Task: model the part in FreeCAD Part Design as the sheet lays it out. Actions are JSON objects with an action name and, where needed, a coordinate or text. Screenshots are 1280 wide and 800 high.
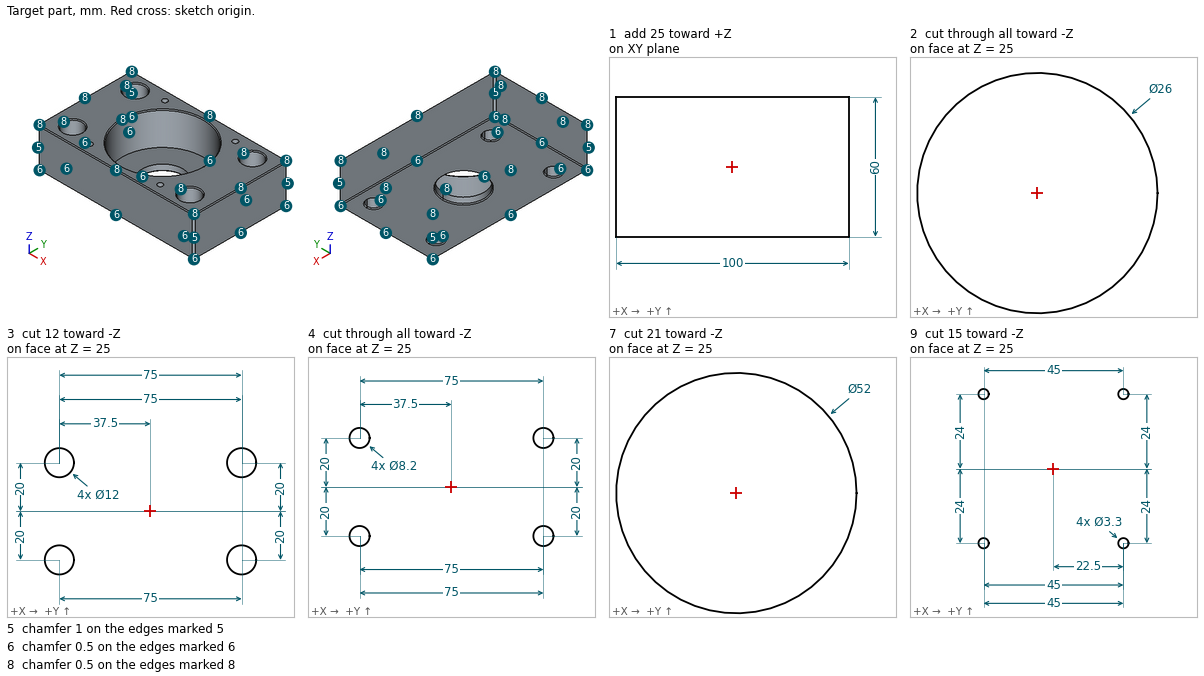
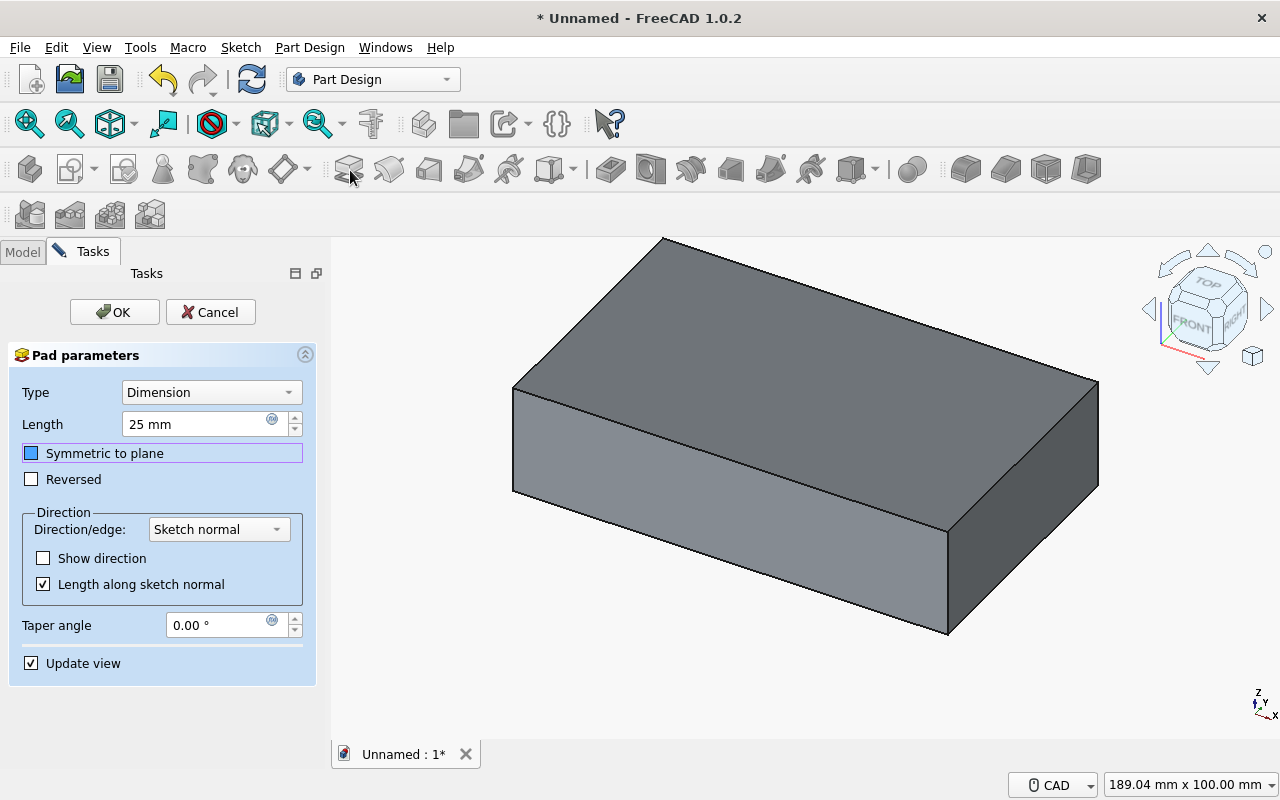
{"action": "left_click", "coordinate": [115, 312]}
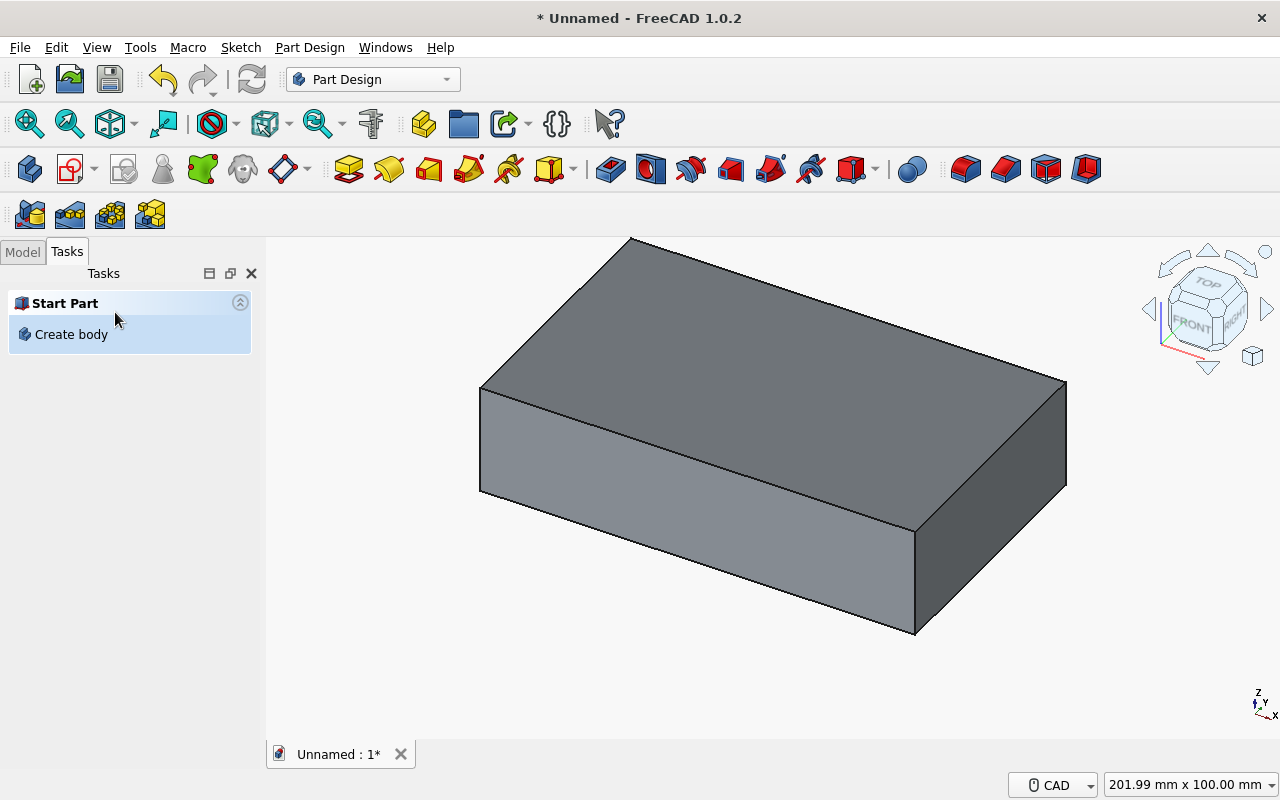
{"action": "left_click", "coordinate": [835, 405]}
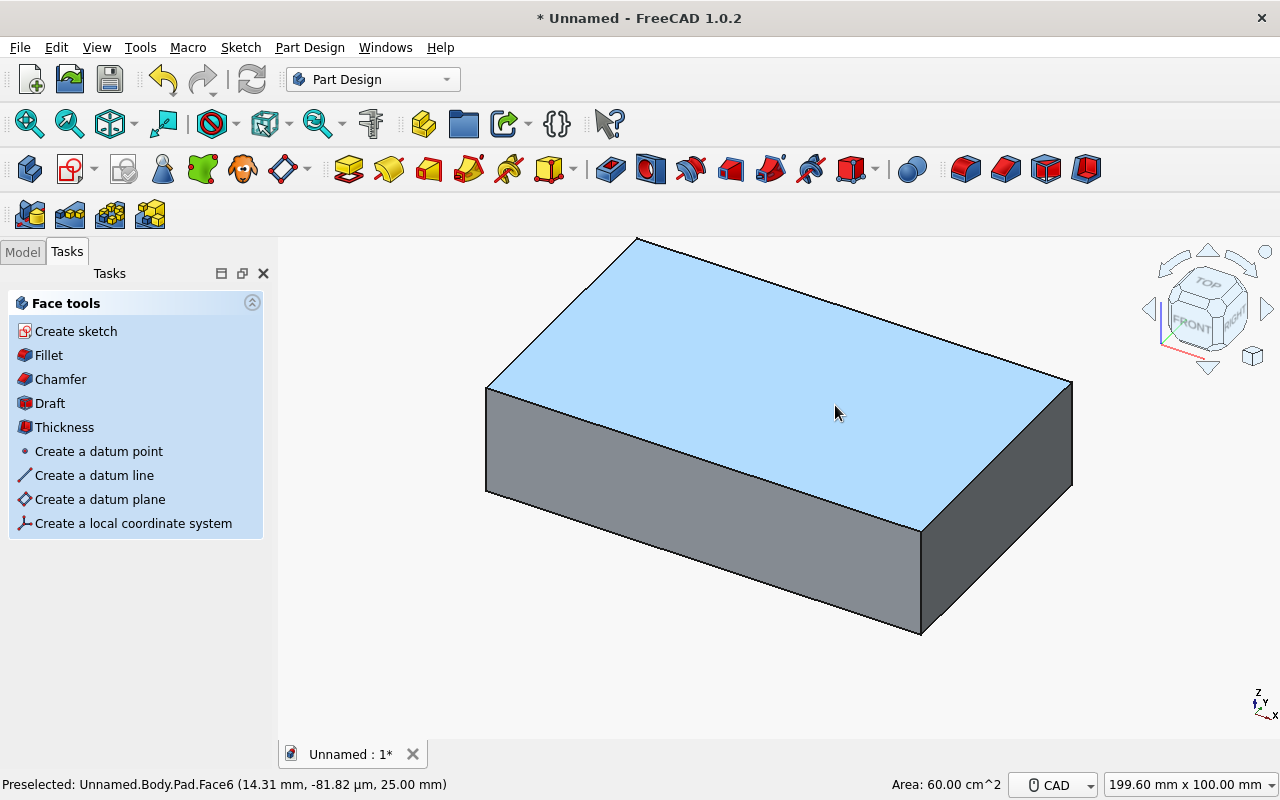
{"action": "left_click", "coordinate": [70, 170]}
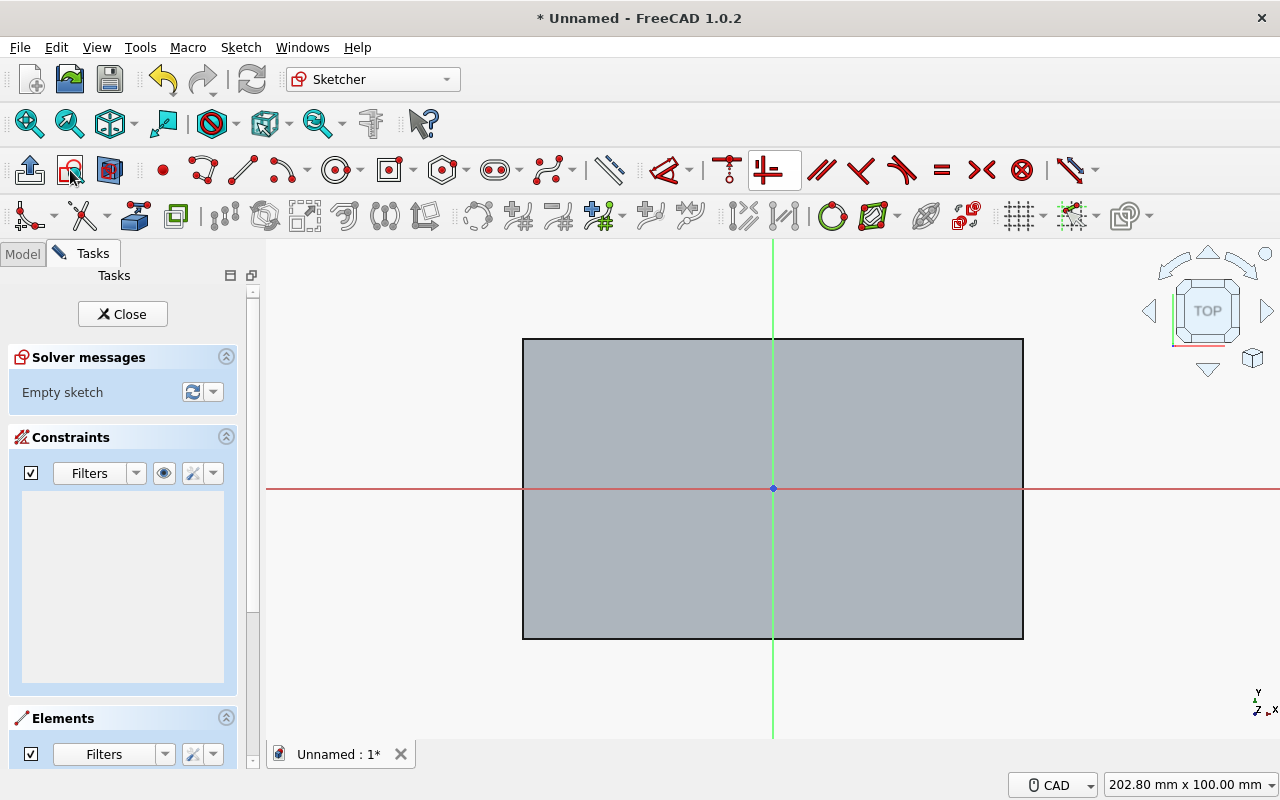
{"action": "scroll", "coordinate": [829, 489], "scroll_direction": "up", "scroll_amount": 4}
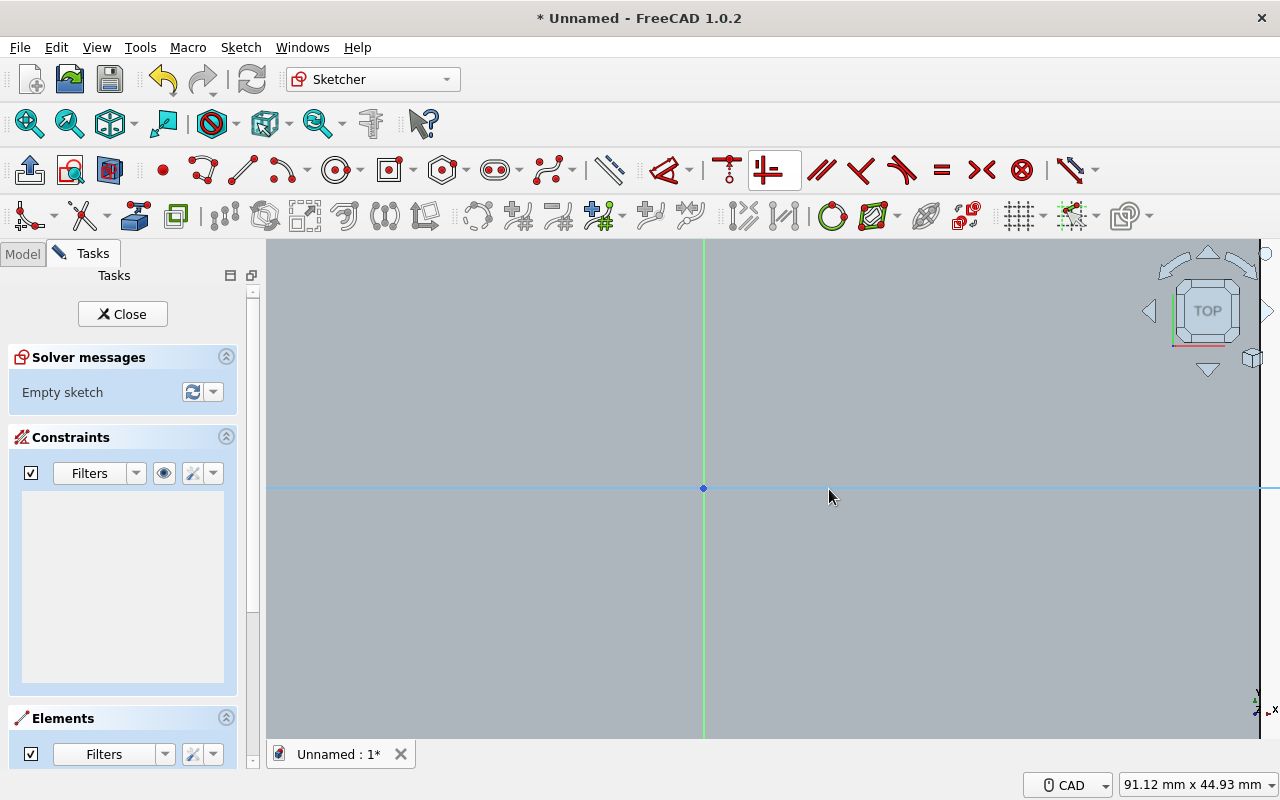
{"action": "left_click", "coordinate": [336, 170]}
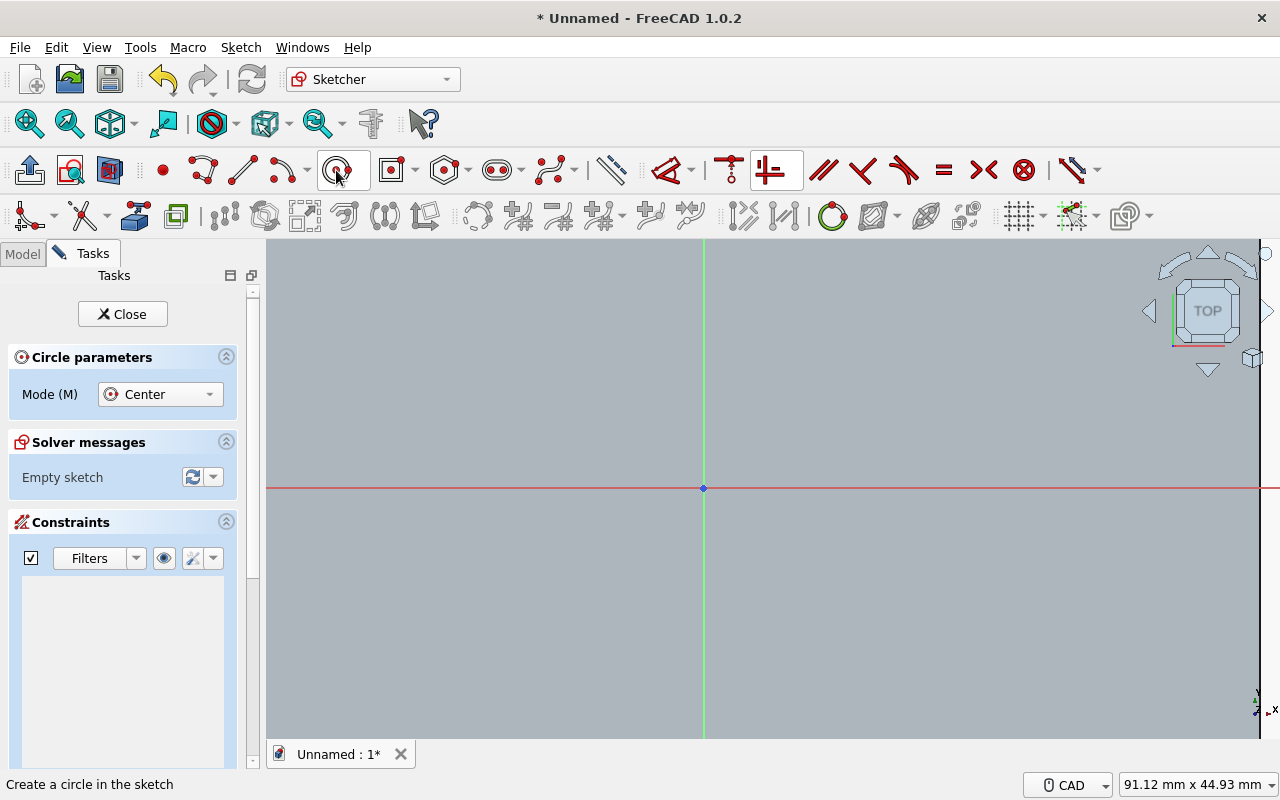
{"action": "left_click", "coordinate": [704, 488]}
{"action": "mouse_move", "coordinate": [806, 386]}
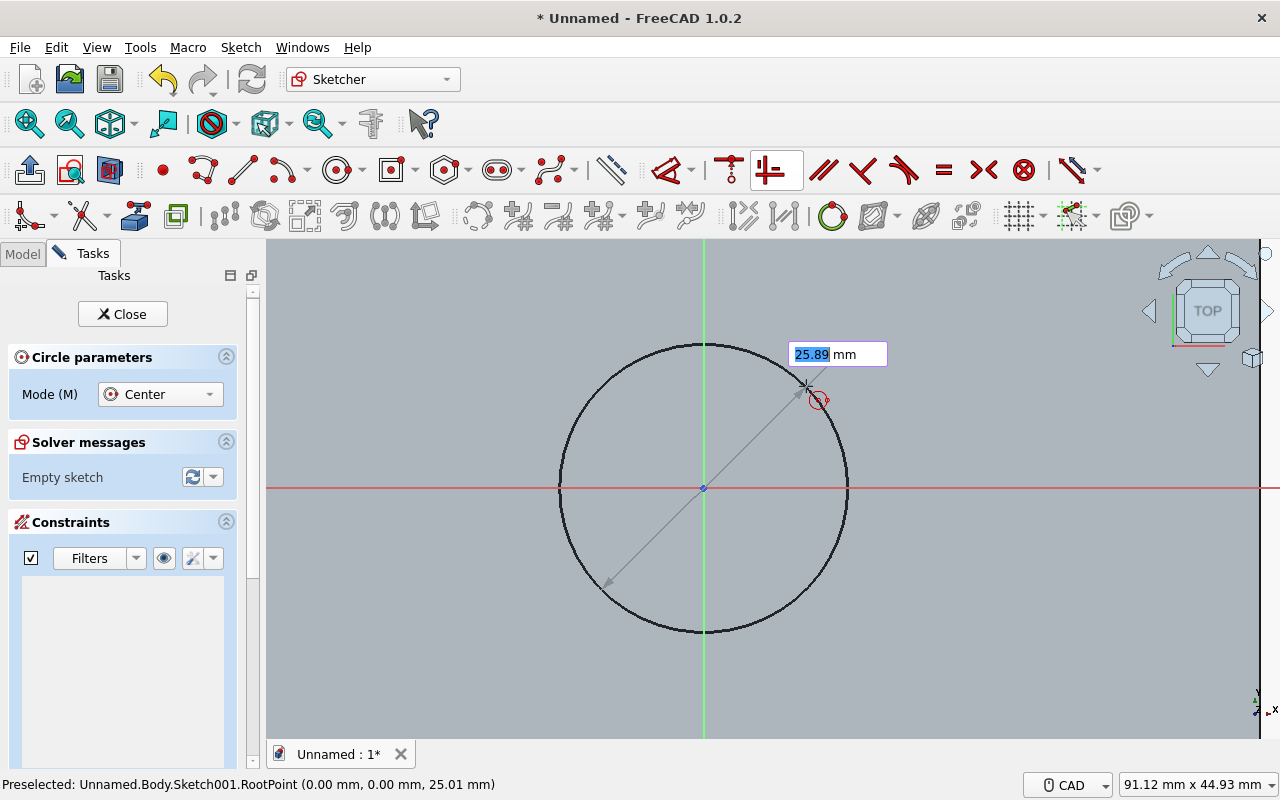
{"action": "type", "text": "26"}
{"action": "key", "text": "Return"}
{"action": "key", "text": "Escape"}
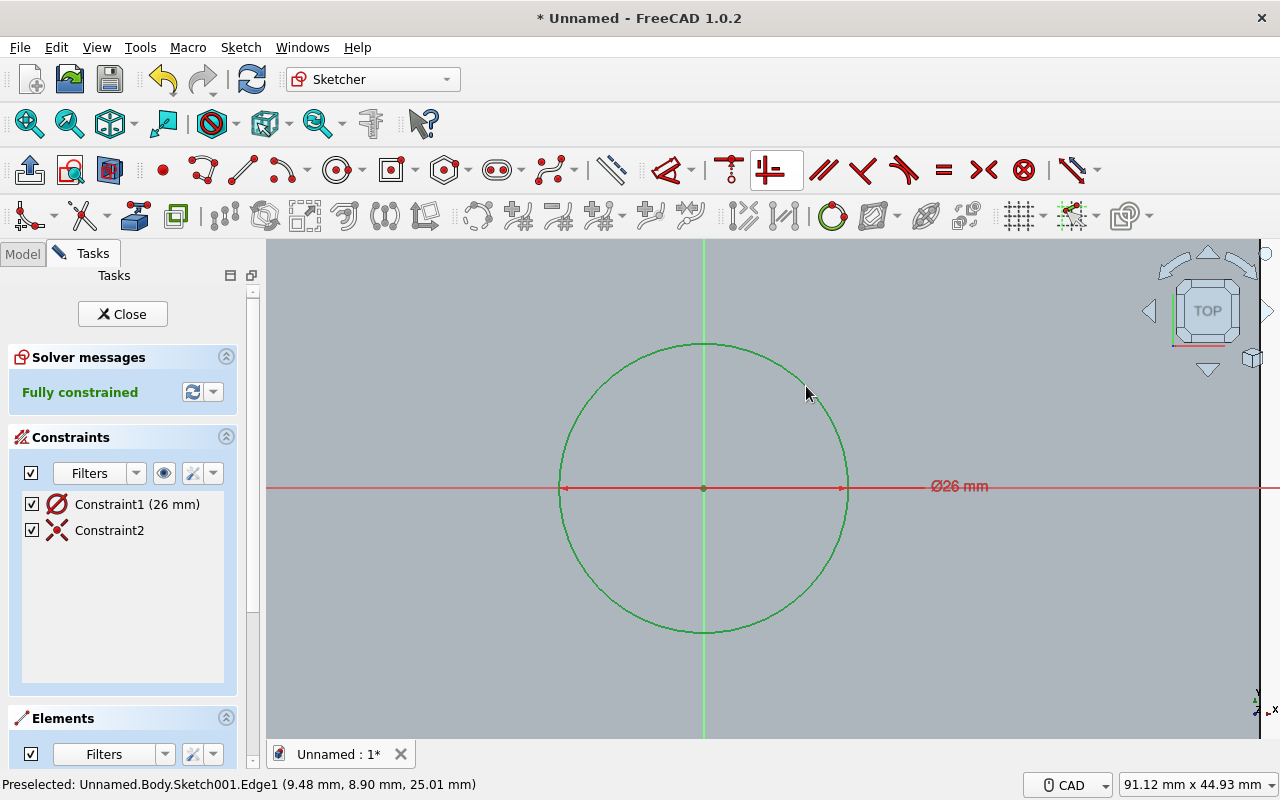
{"action": "left_click", "coordinate": [123, 314]}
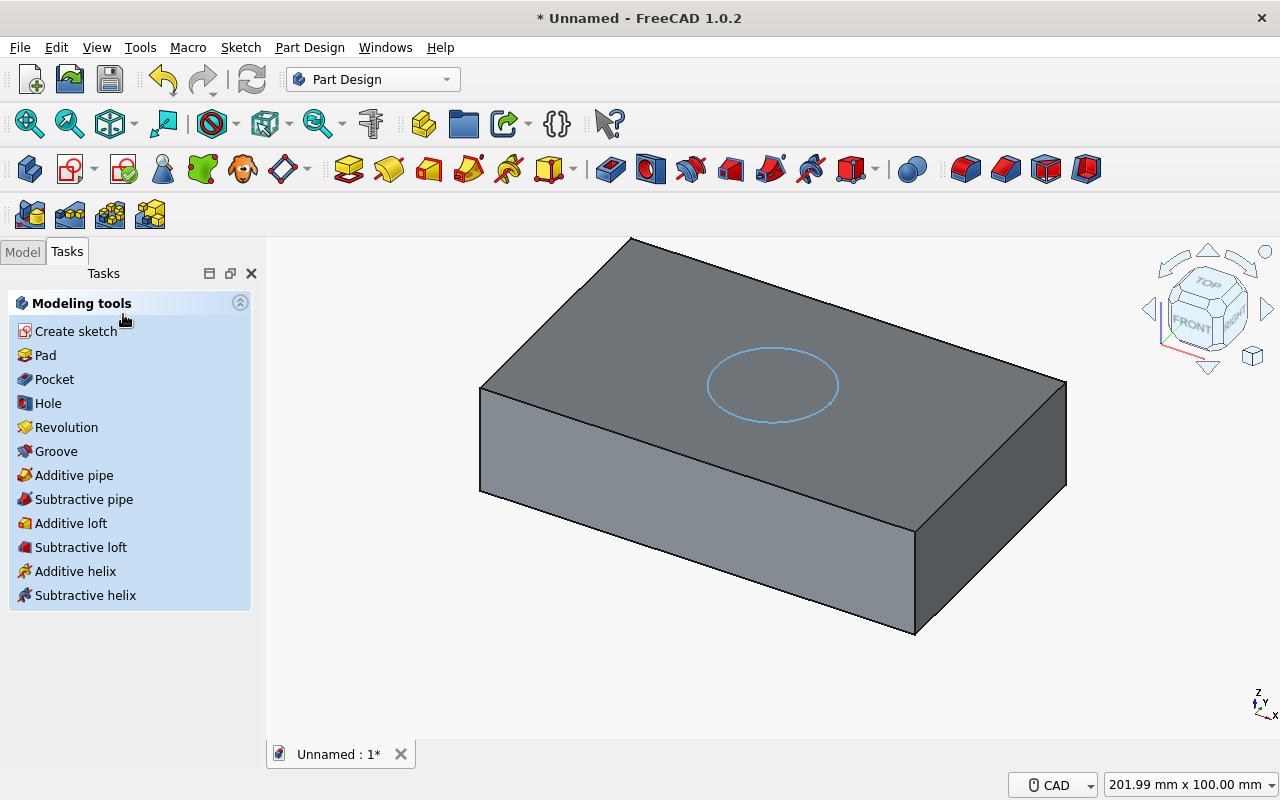
{"action": "left_click", "coordinate": [612, 170]}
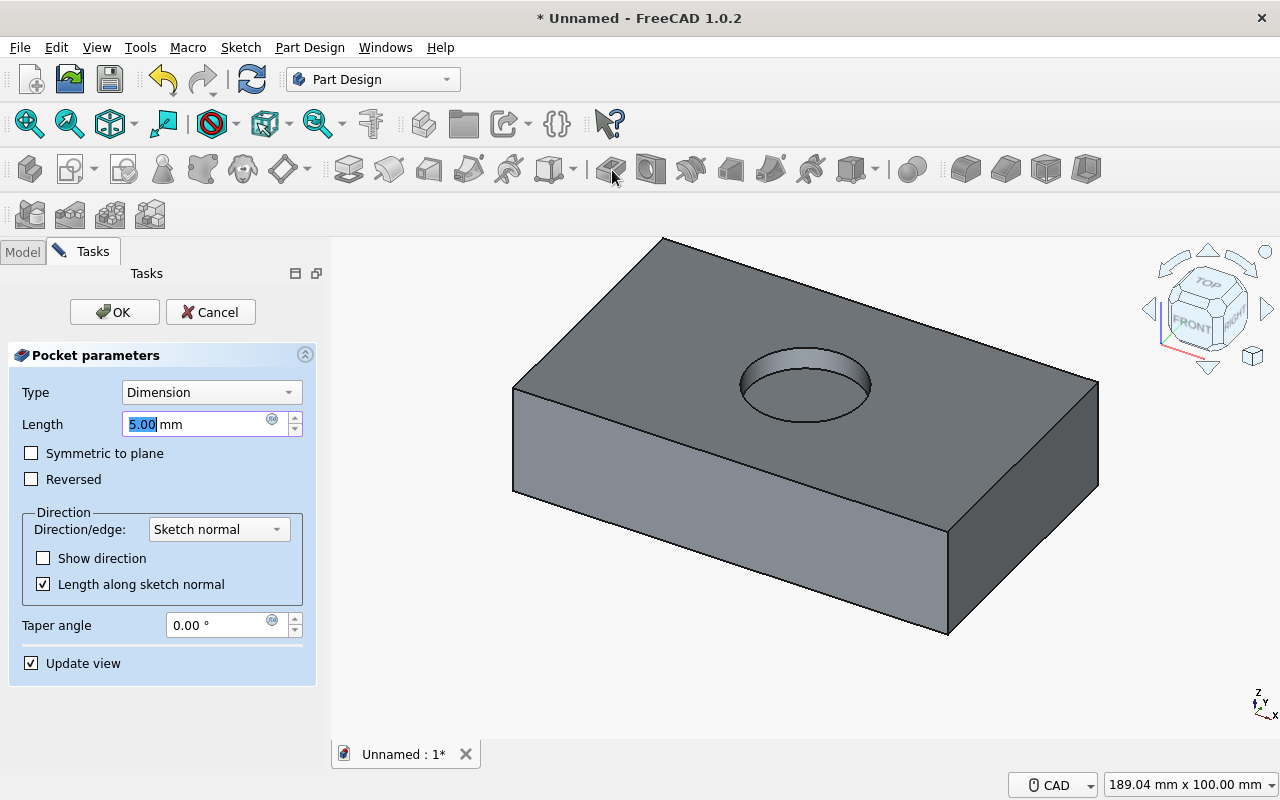
{"action": "left_click", "coordinate": [212, 392]}